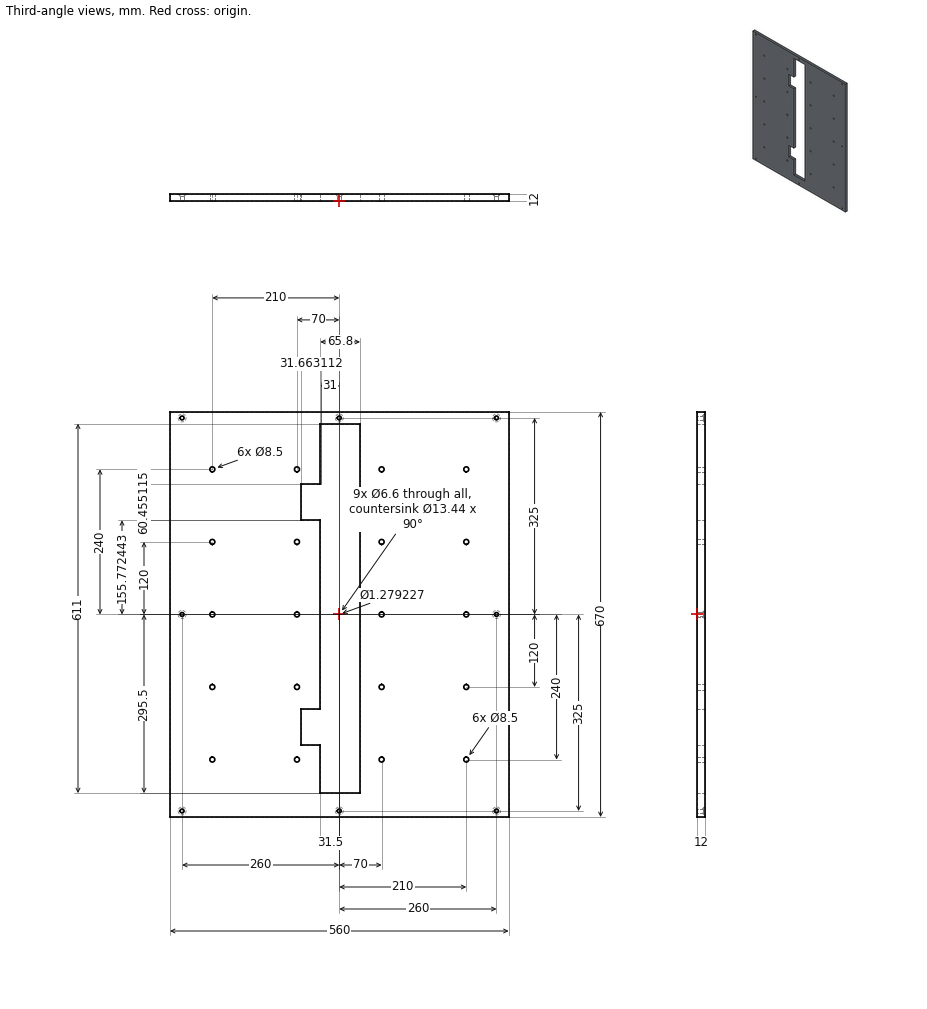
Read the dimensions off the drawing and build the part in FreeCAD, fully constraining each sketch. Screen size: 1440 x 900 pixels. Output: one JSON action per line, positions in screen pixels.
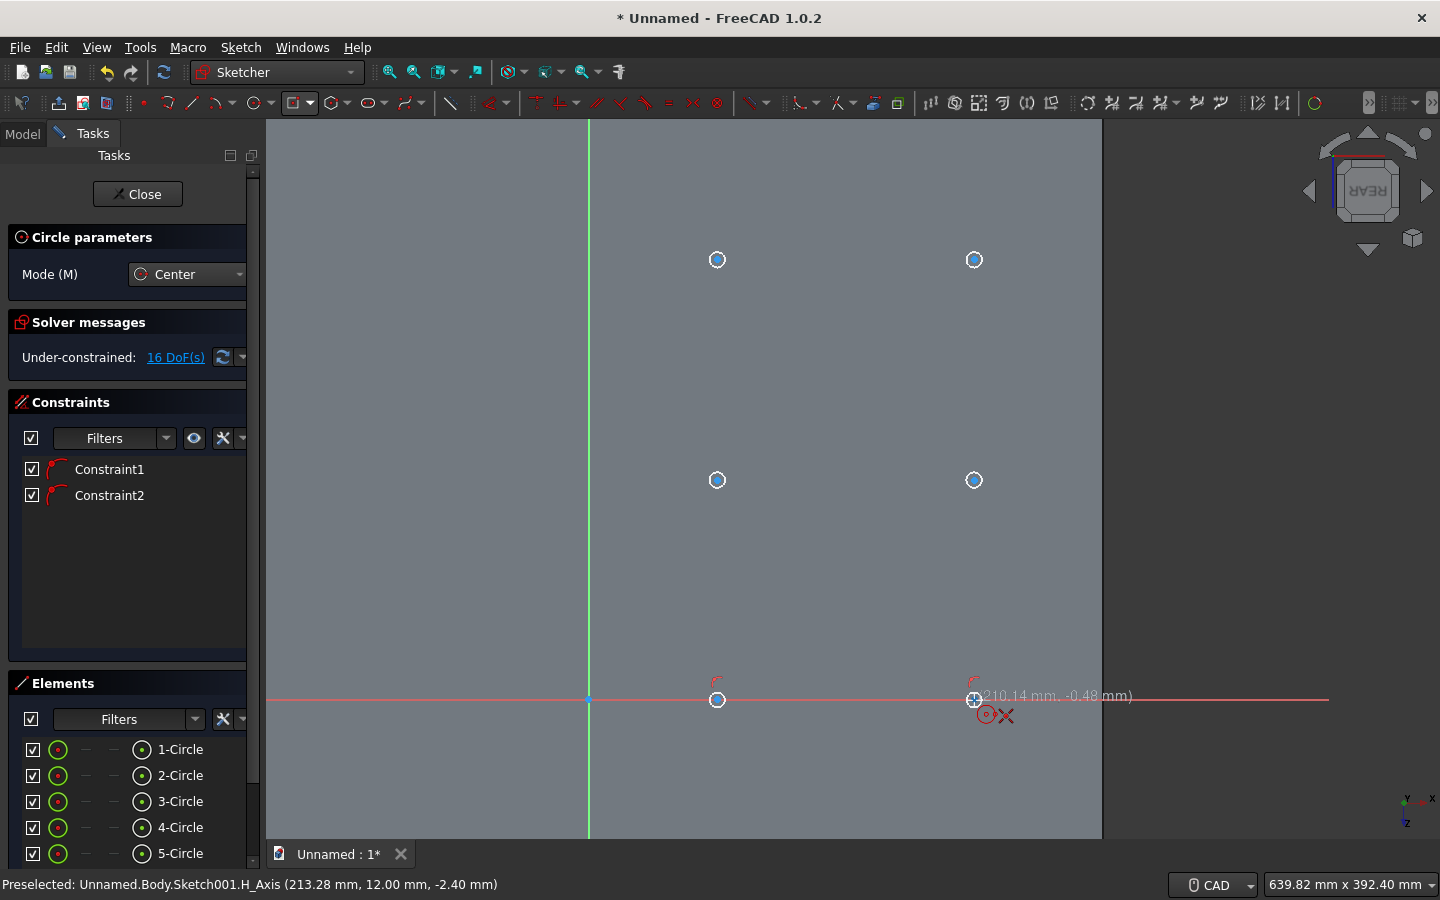
{"action": "scroll", "coordinate": [589, 700], "scroll_direction": "up", "scroll_amount": 15}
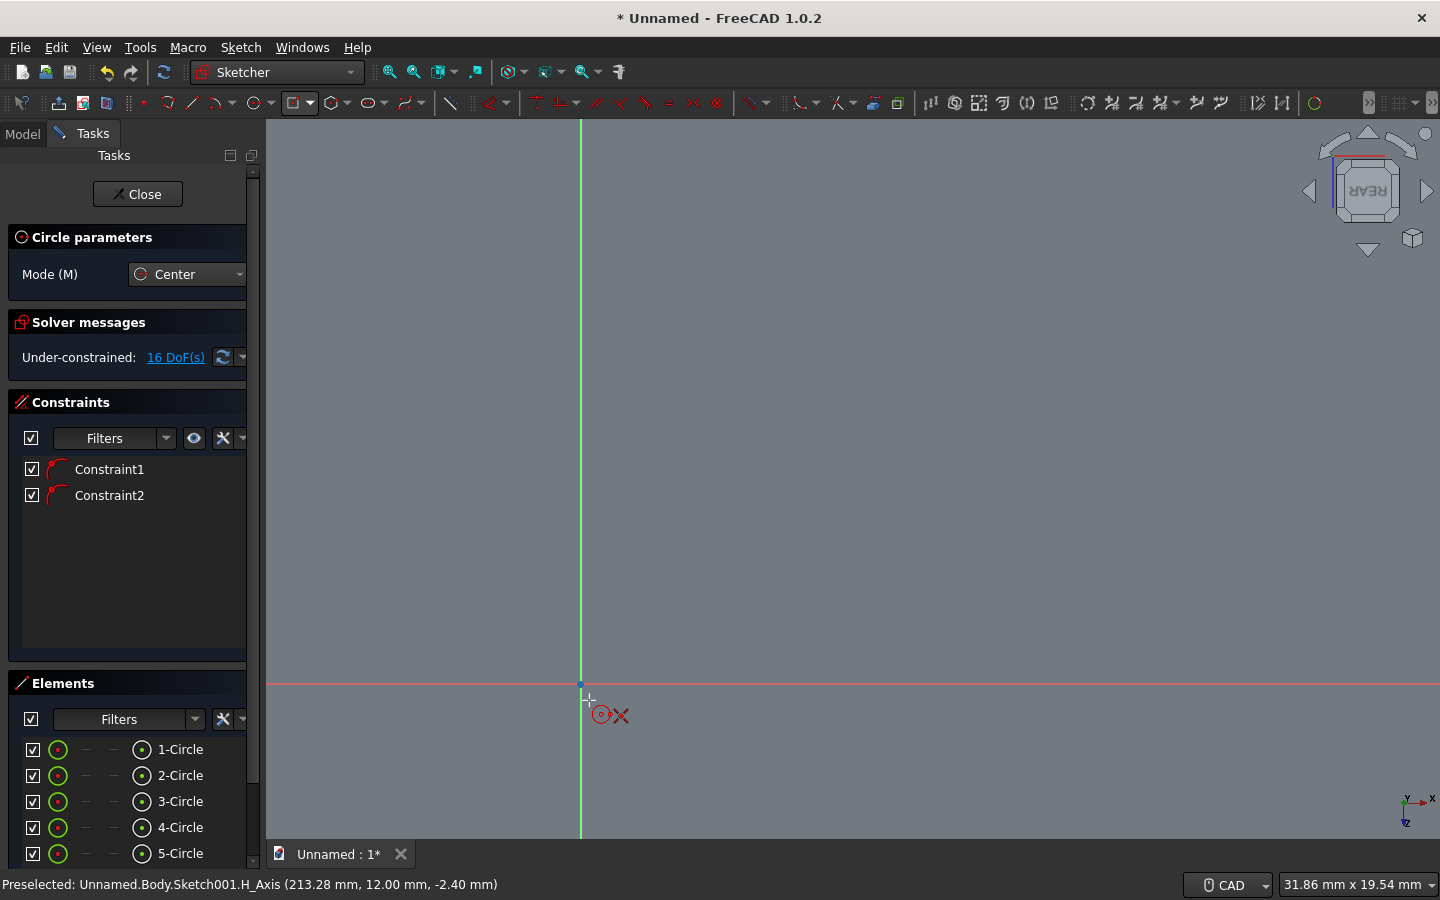
{"action": "scroll", "coordinate": [589, 700], "scroll_direction": "down", "scroll_amount": 15}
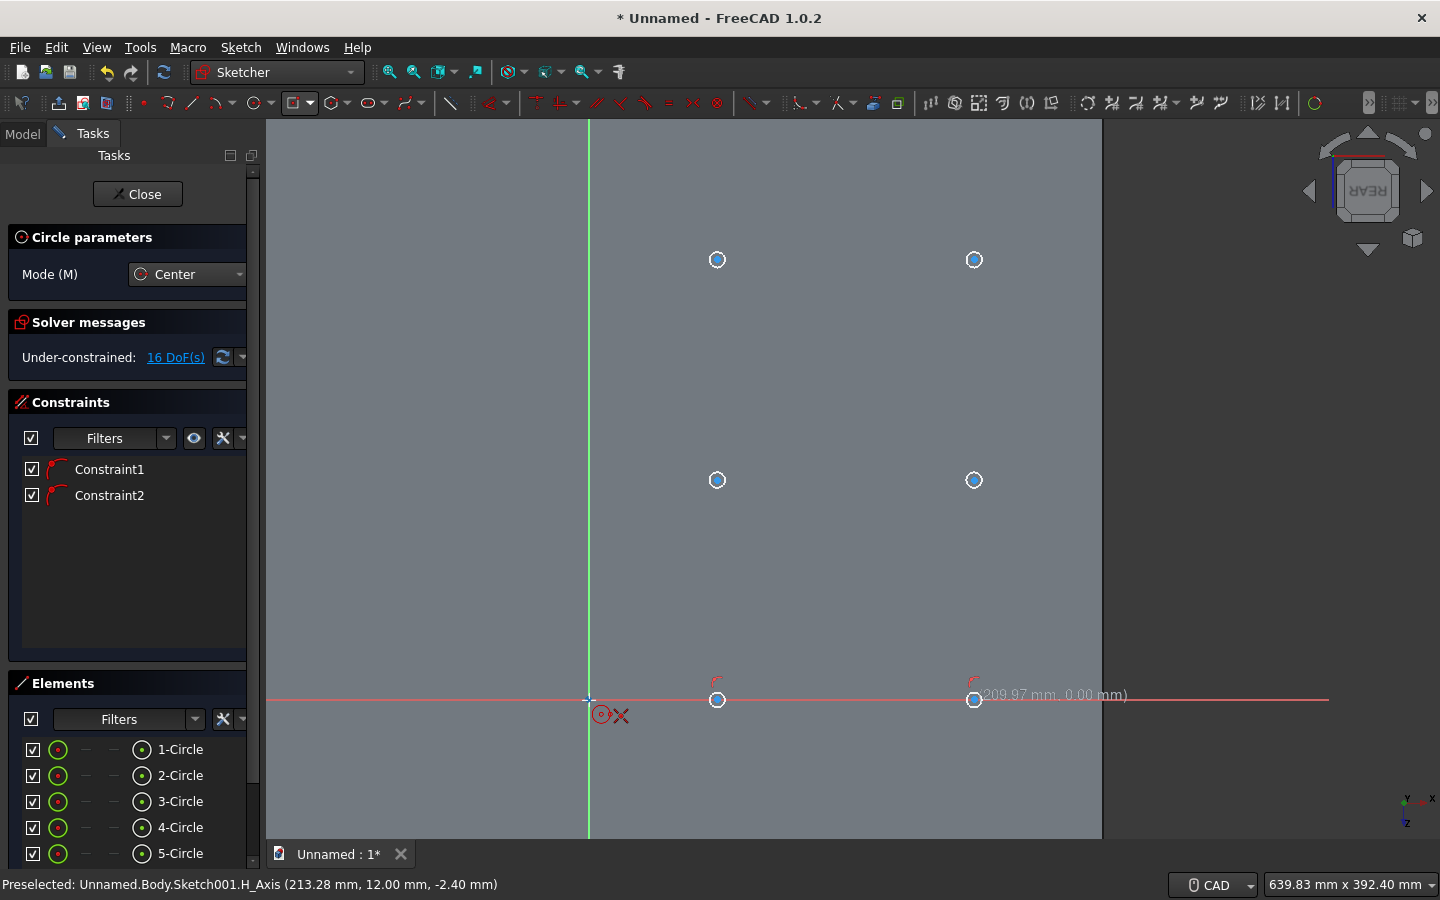
{"action": "left_click", "coordinate": [589, 700]}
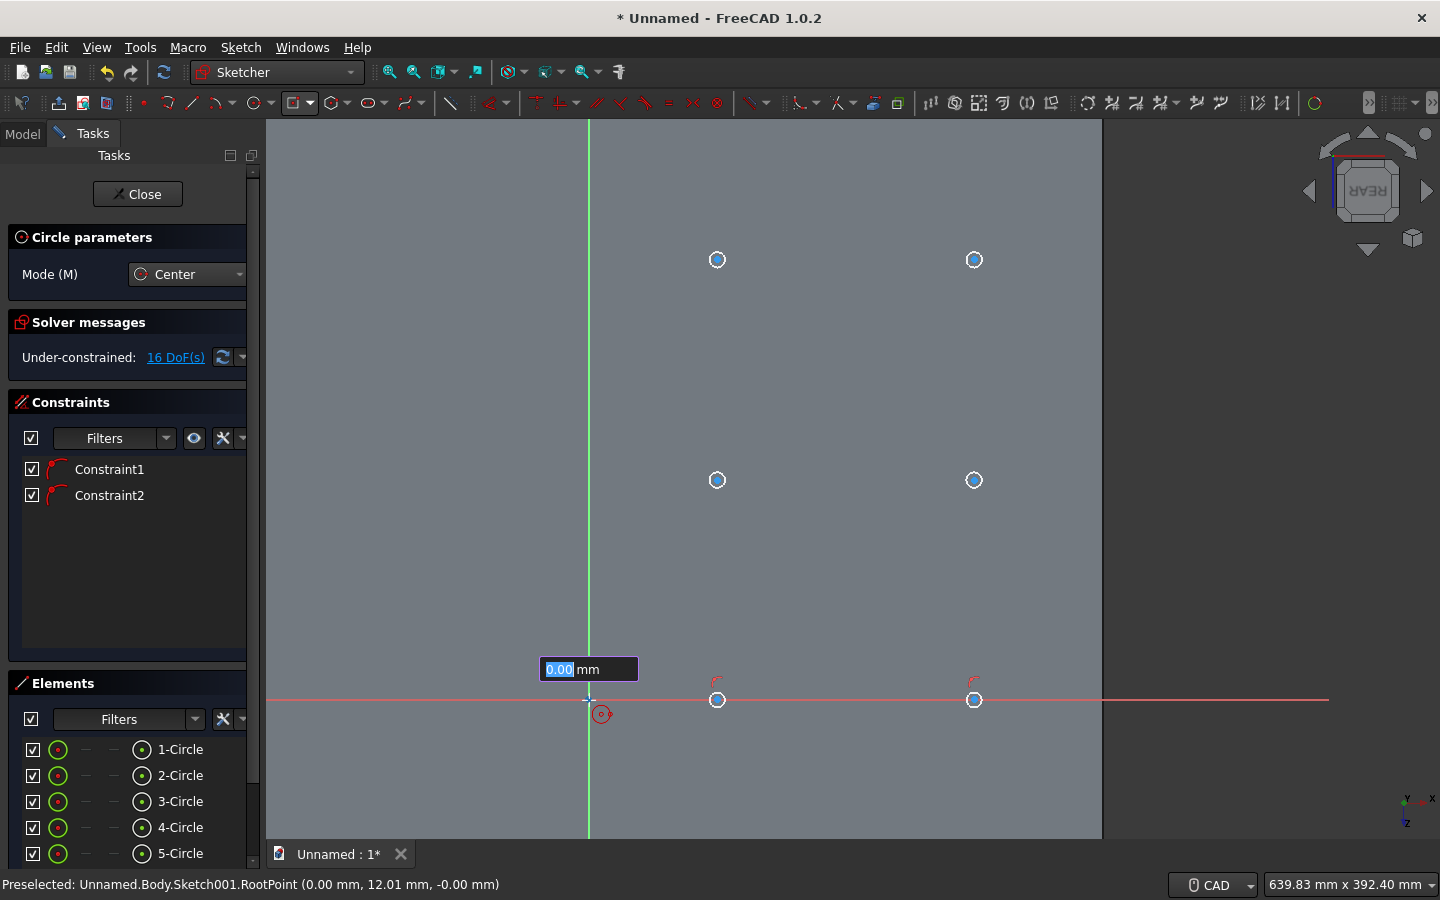
{"action": "scroll", "coordinate": [590, 699], "scroll_direction": "up", "scroll_amount": 15}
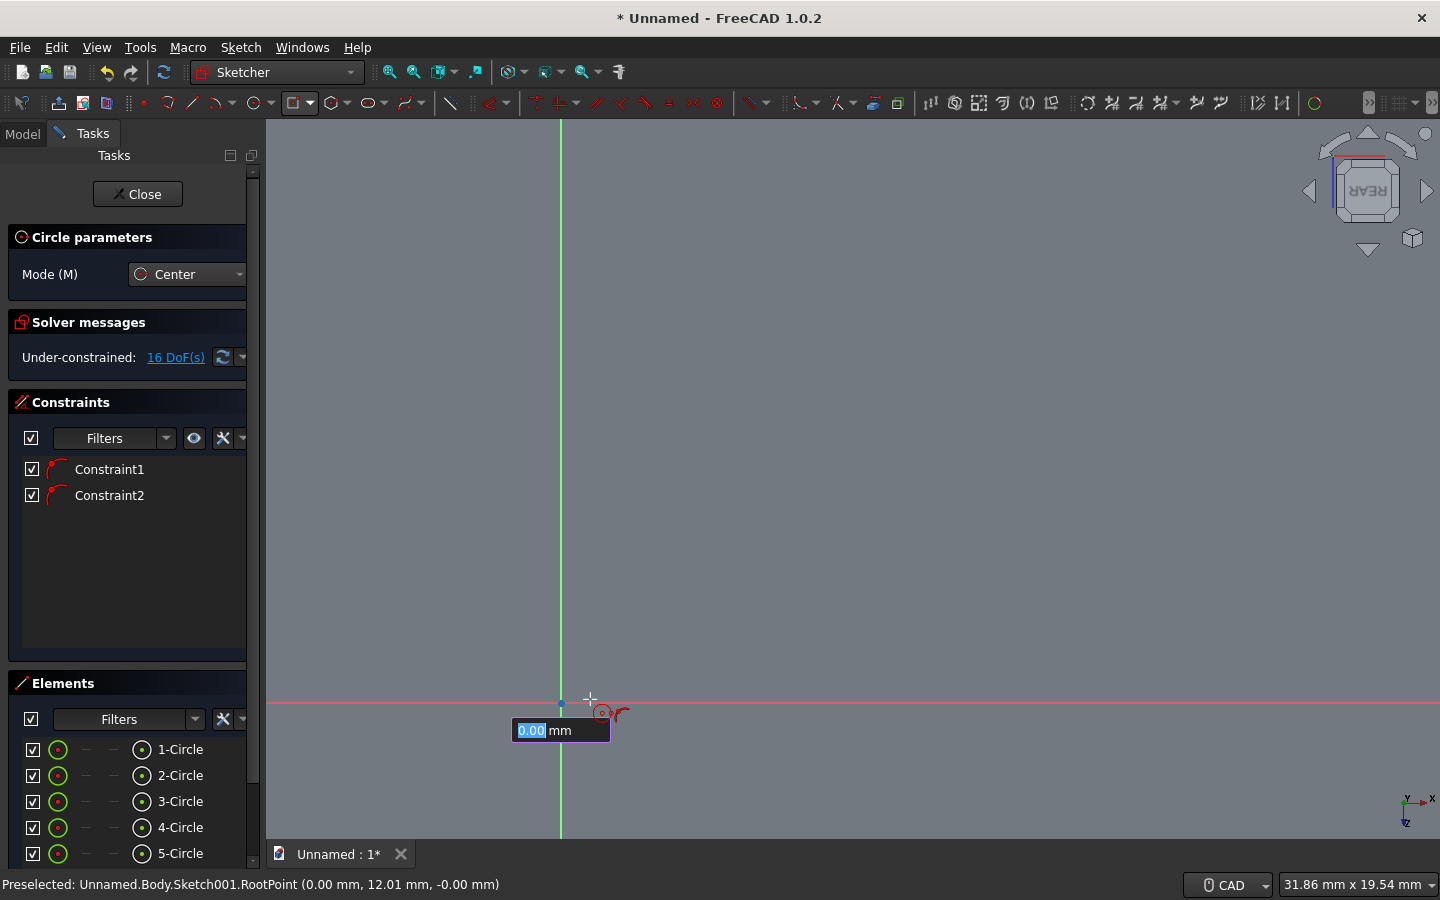
{"action": "left_click", "coordinate": [578, 687]}
{"action": "key", "text": "Escape"}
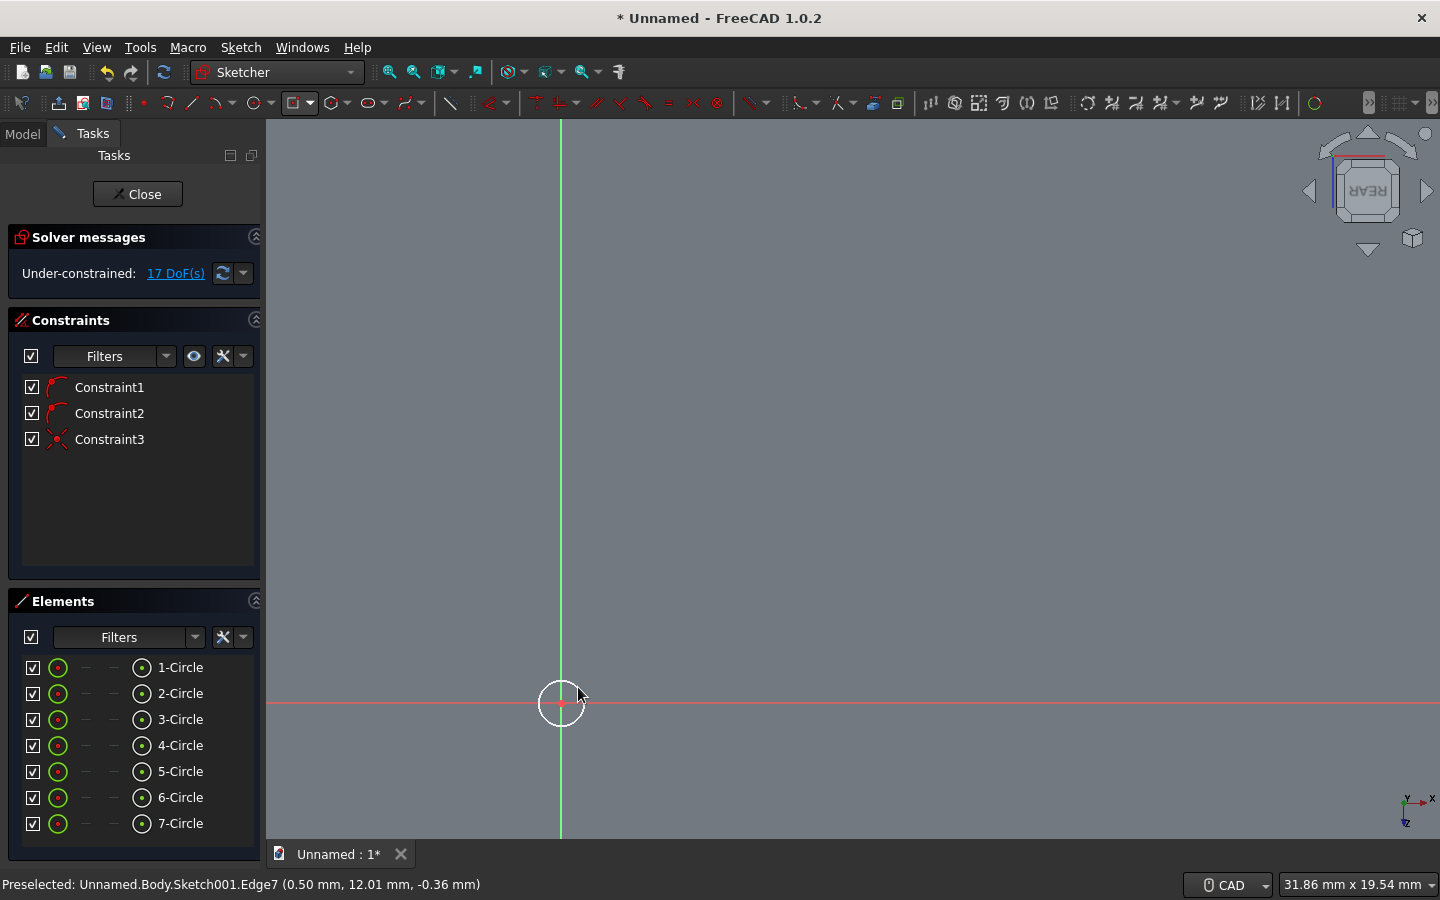
{"action": "scroll", "coordinate": [590, 699], "scroll_direction": "down", "scroll_amount": 15}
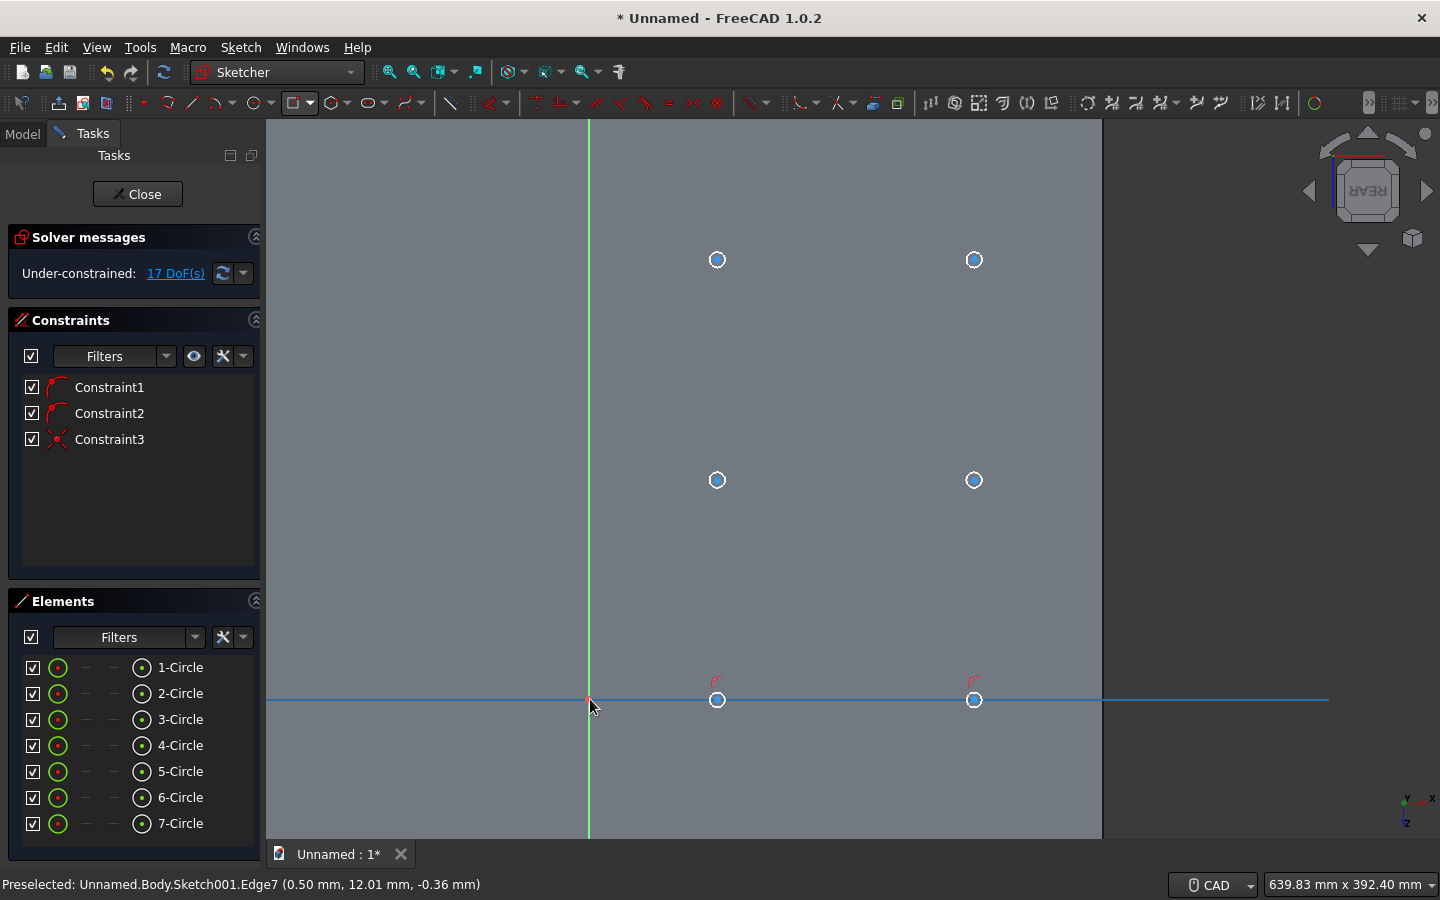
{"action": "scroll", "coordinate": [980, 254], "scroll_direction": "up", "scroll_amount": 3}